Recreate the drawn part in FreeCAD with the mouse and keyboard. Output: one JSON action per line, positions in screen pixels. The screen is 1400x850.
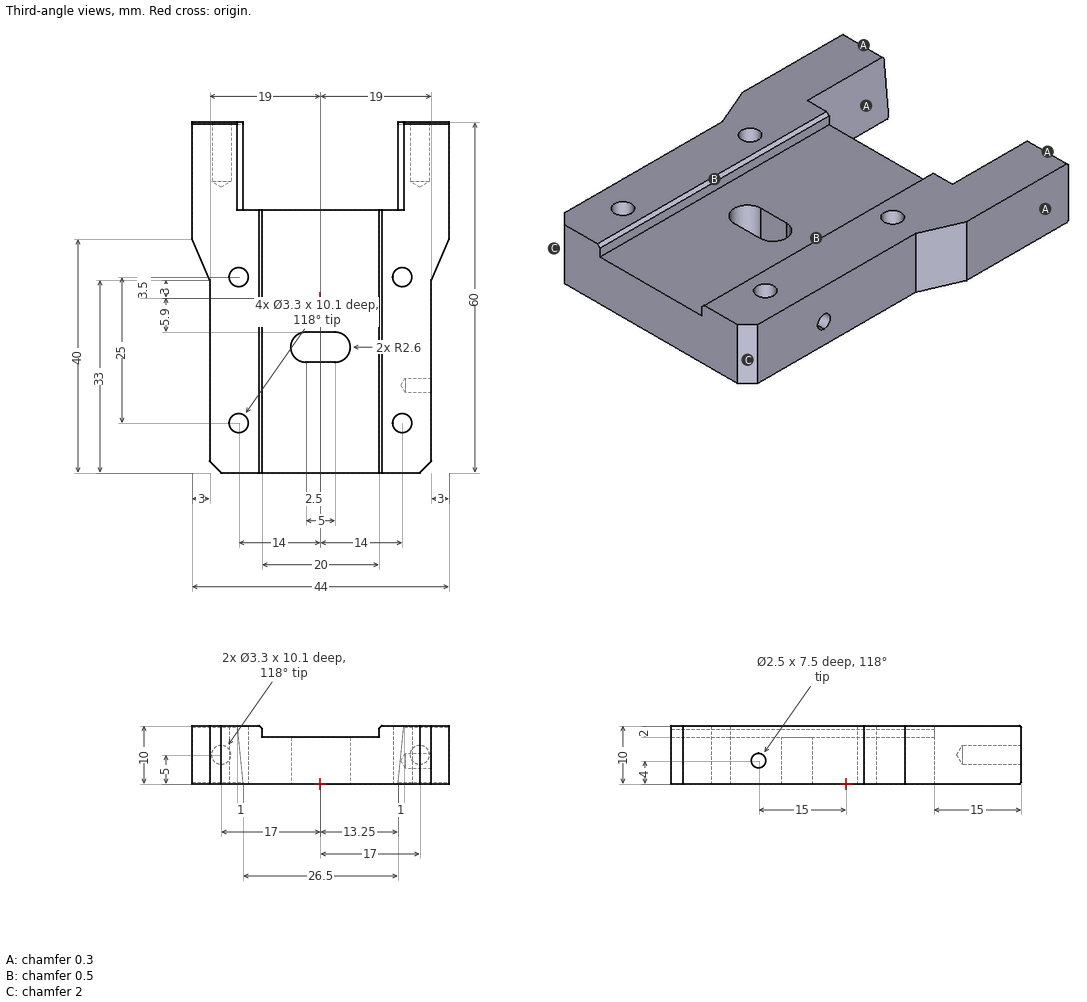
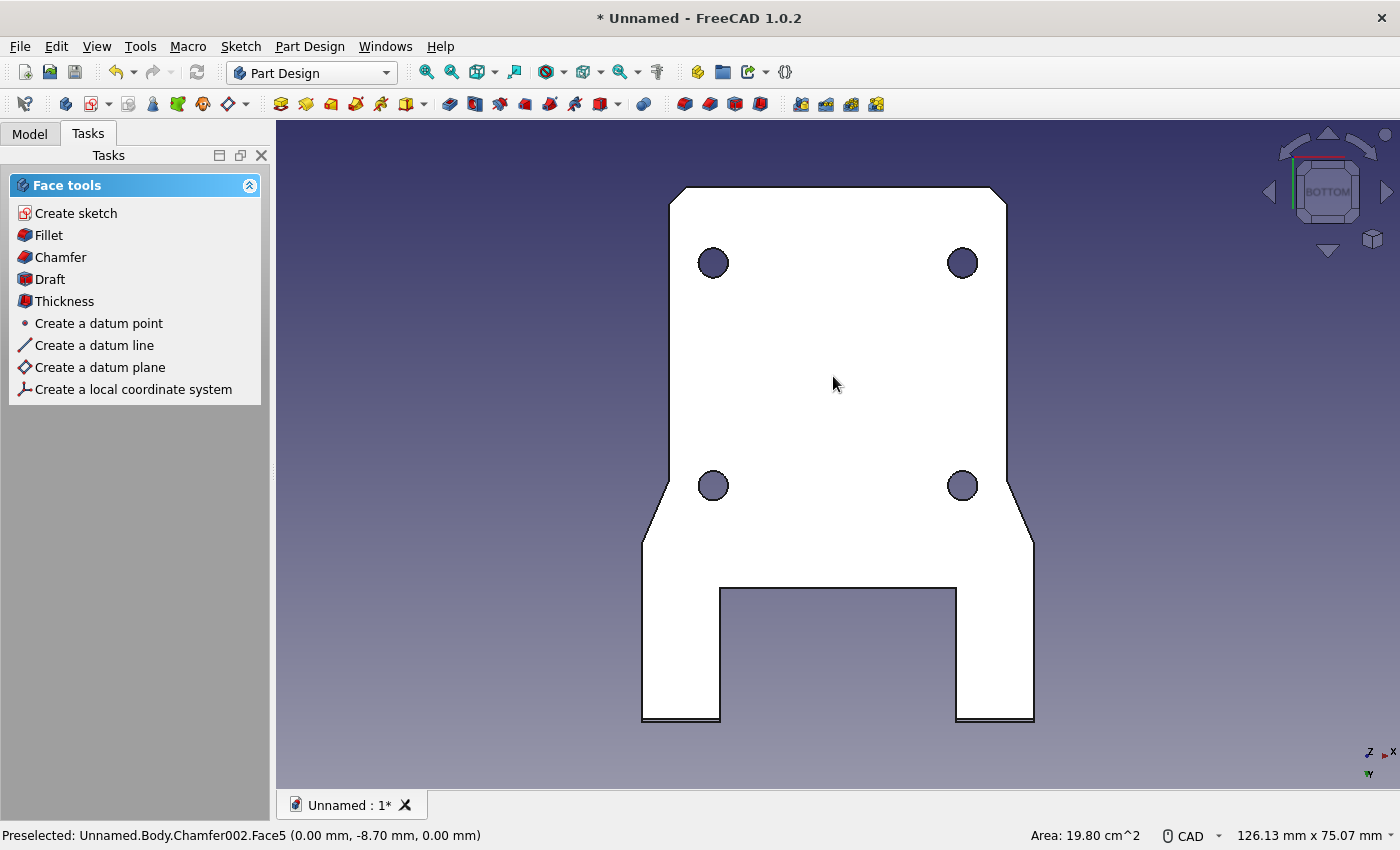
{"action": "left_click", "coordinate": [90, 104]}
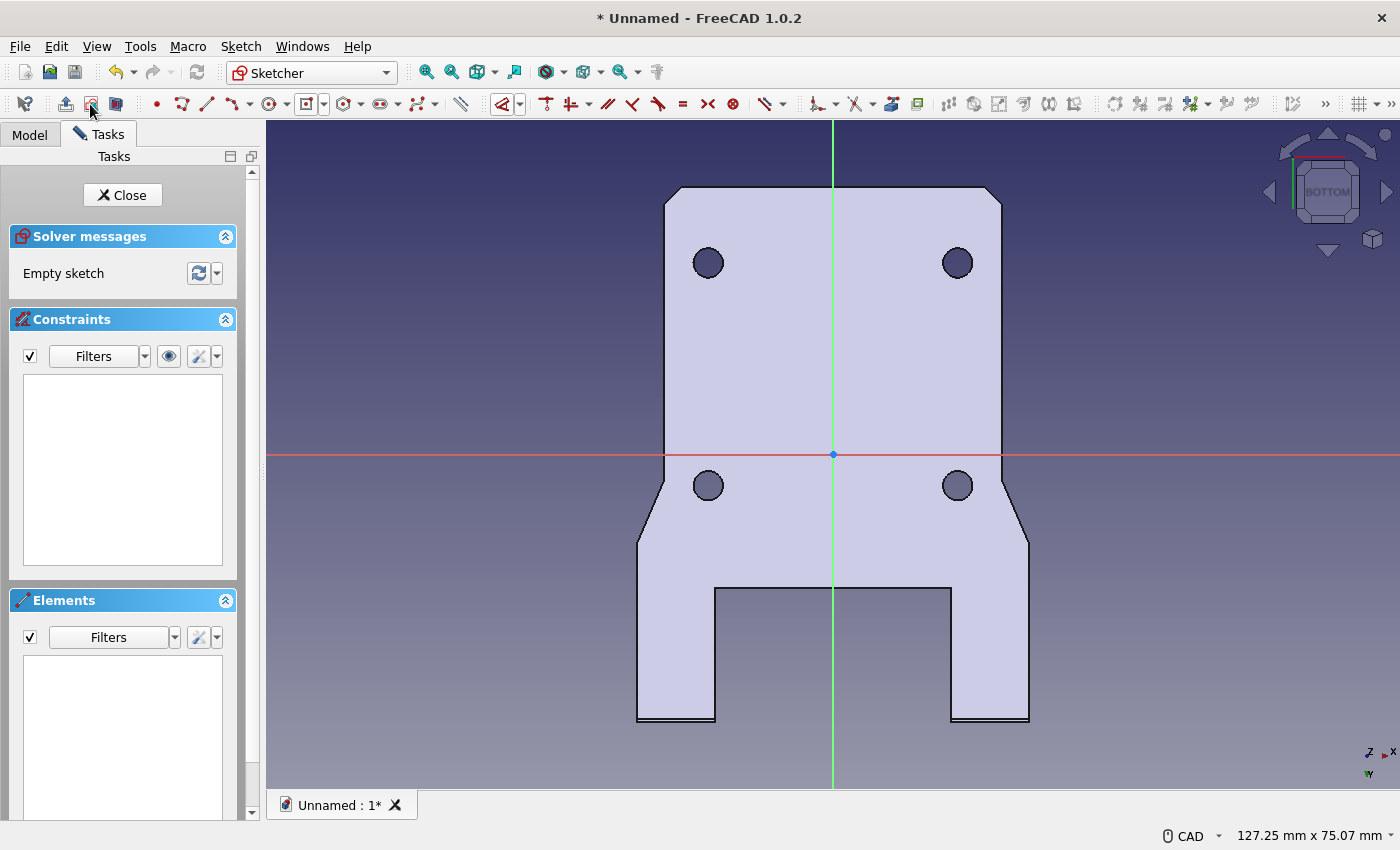
{"action": "scroll", "coordinate": [855, 389], "scroll_direction": "up", "scroll_amount": 7}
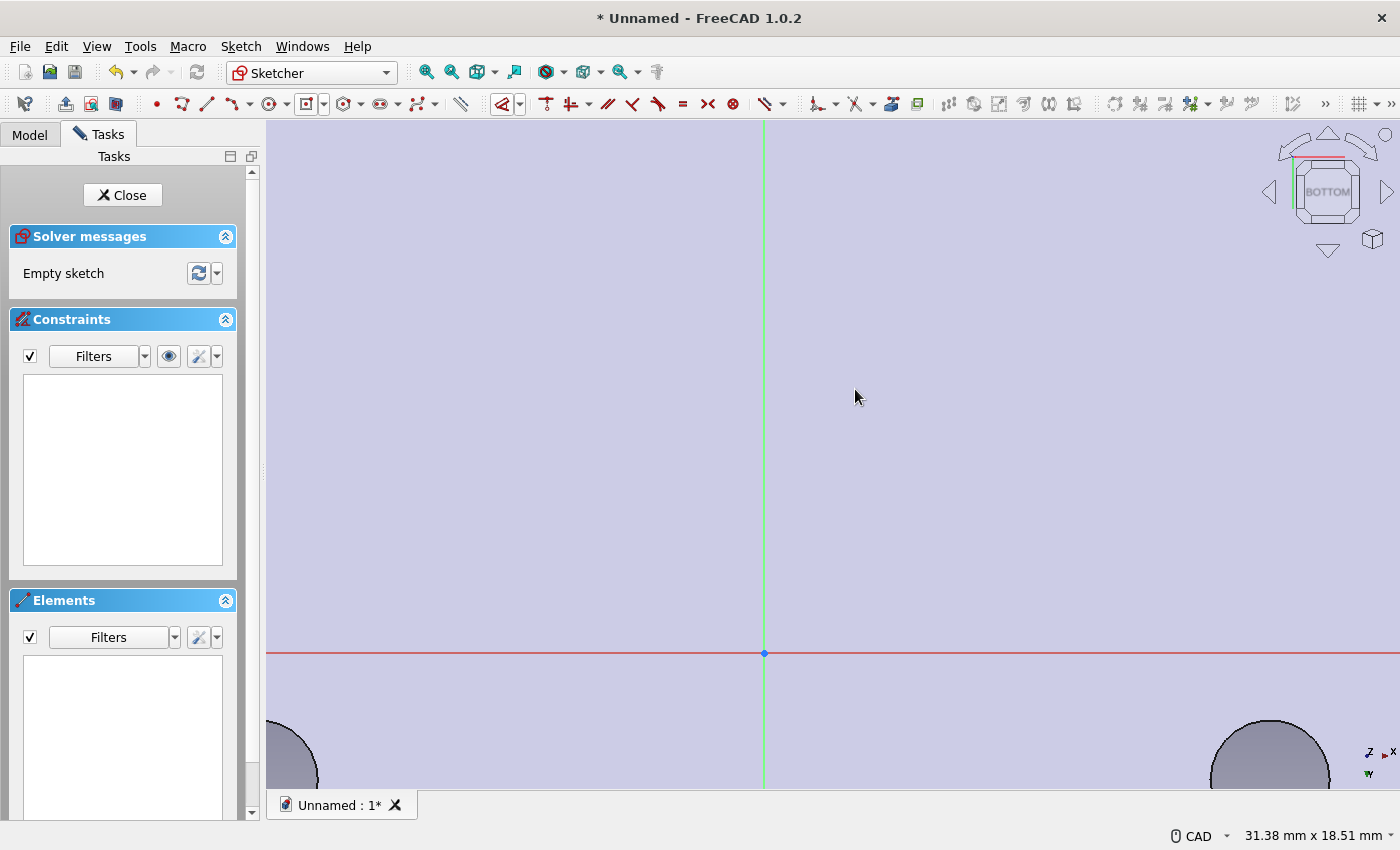
{"action": "left_click", "coordinate": [380, 104]}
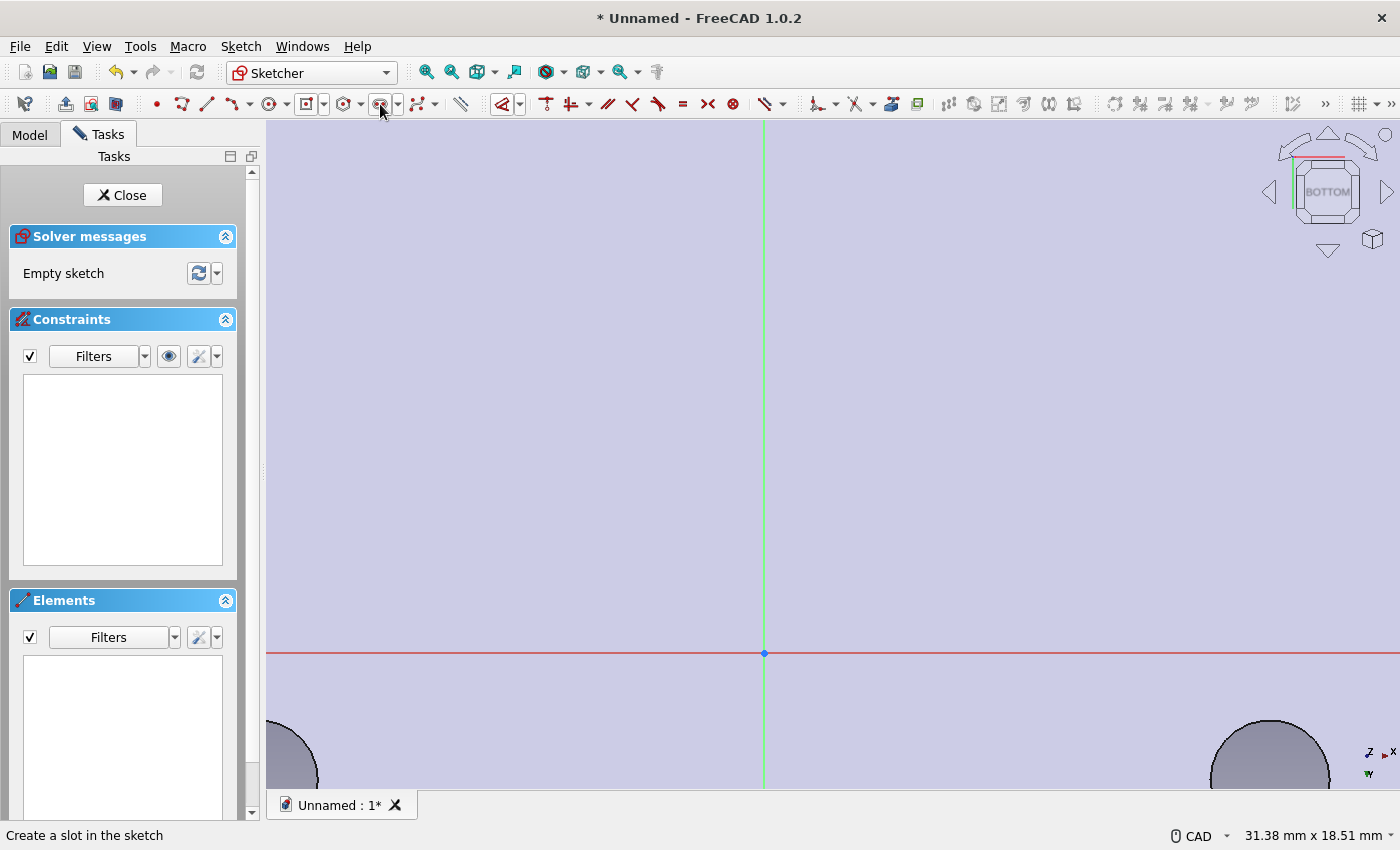
{"action": "left_click", "coordinate": [674, 346]}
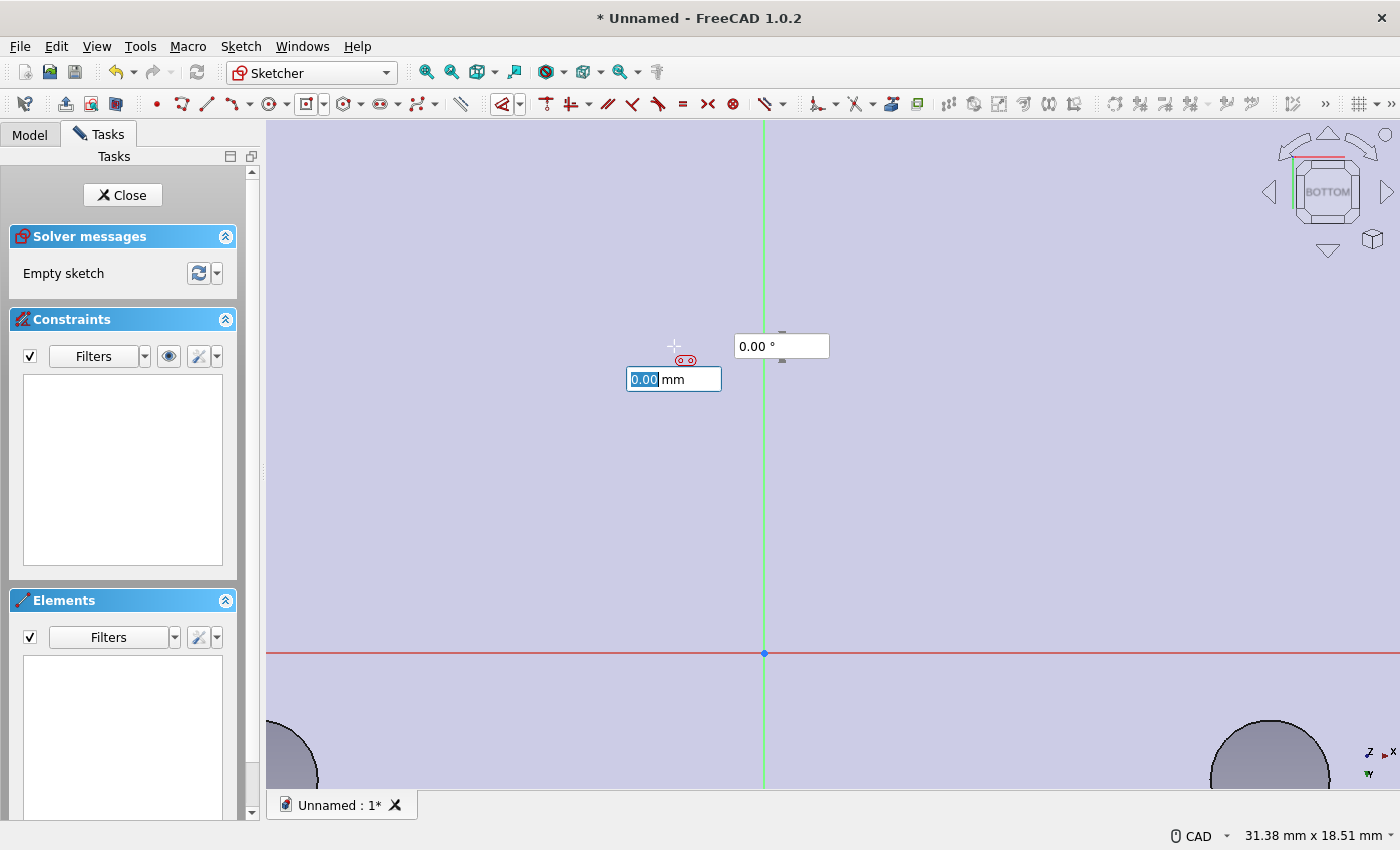
{"action": "left_click", "coordinate": [855, 346]}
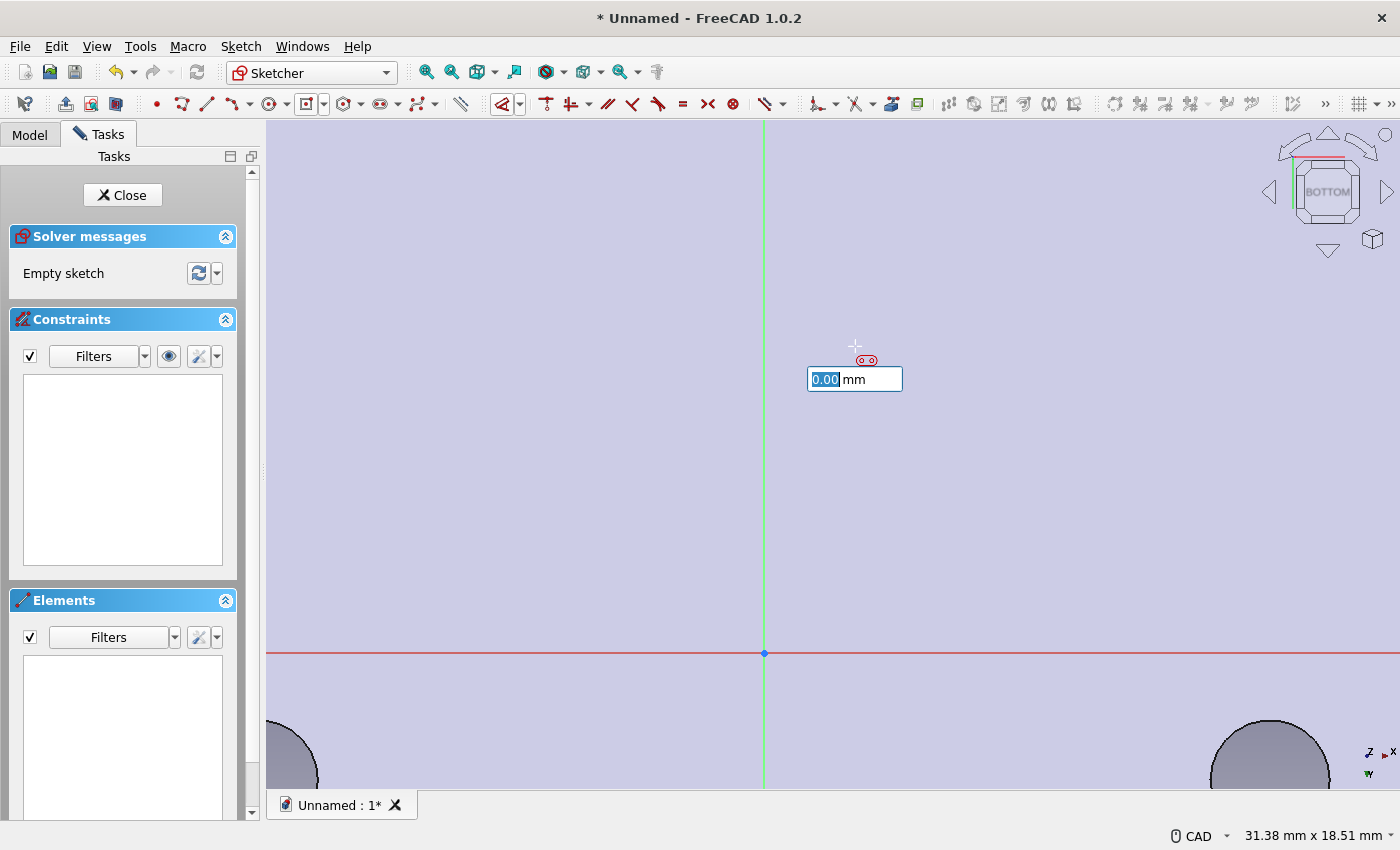
{"action": "left_click", "coordinate": [737, 440]}
{"action": "key", "text": "Escape"}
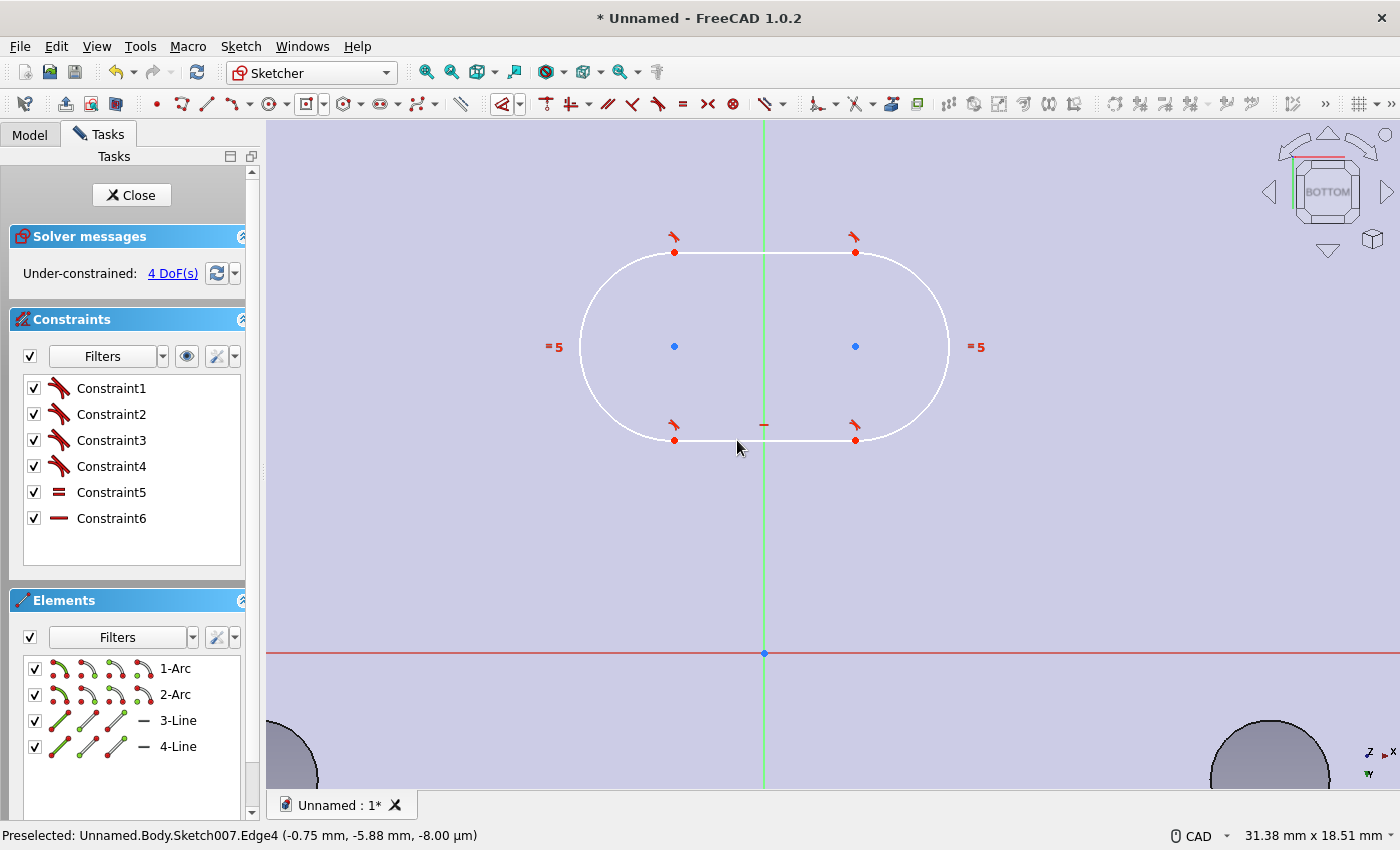
{"action": "left_click", "coordinate": [598, 292]}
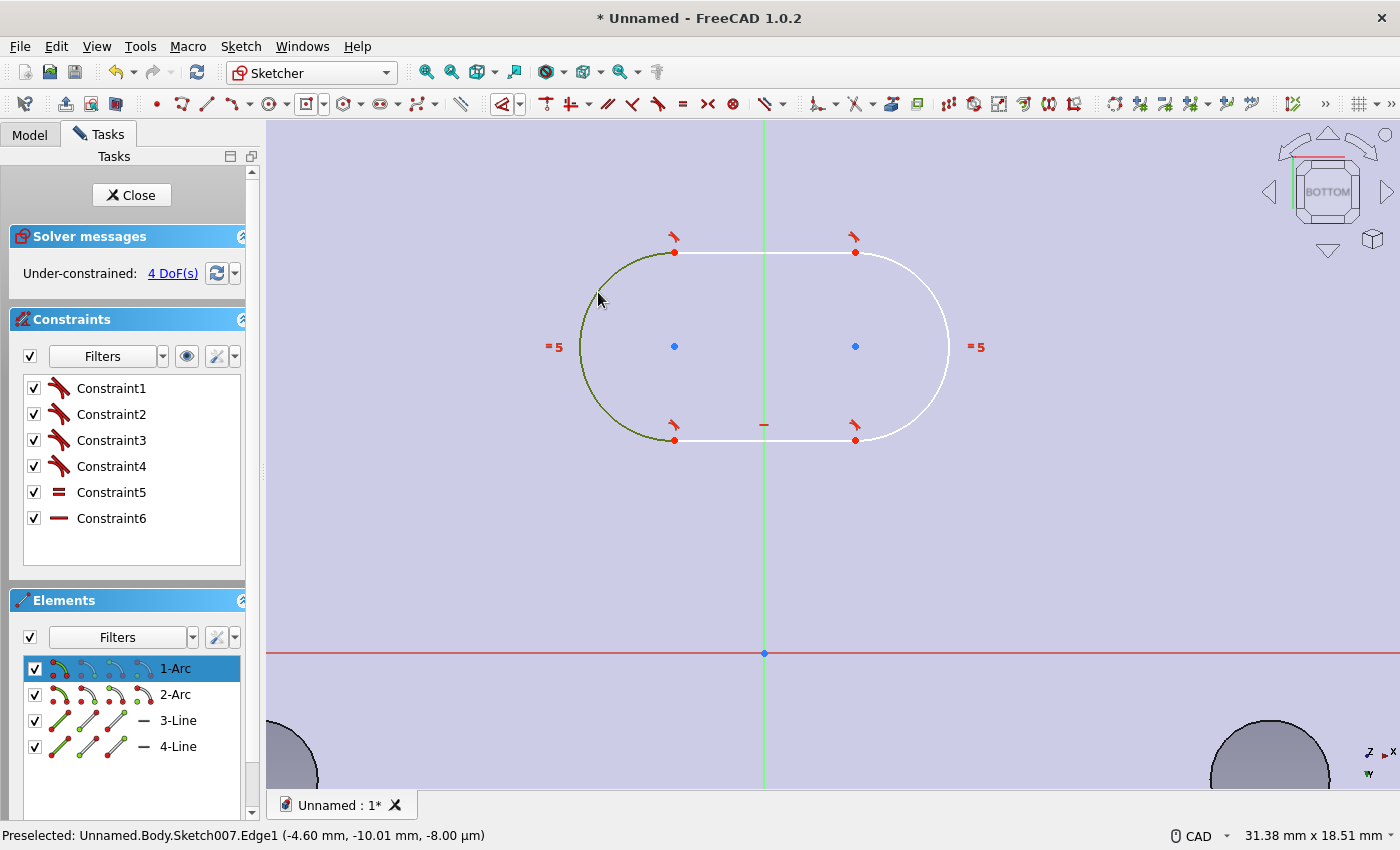
{"action": "left_click", "coordinate": [520, 104]}